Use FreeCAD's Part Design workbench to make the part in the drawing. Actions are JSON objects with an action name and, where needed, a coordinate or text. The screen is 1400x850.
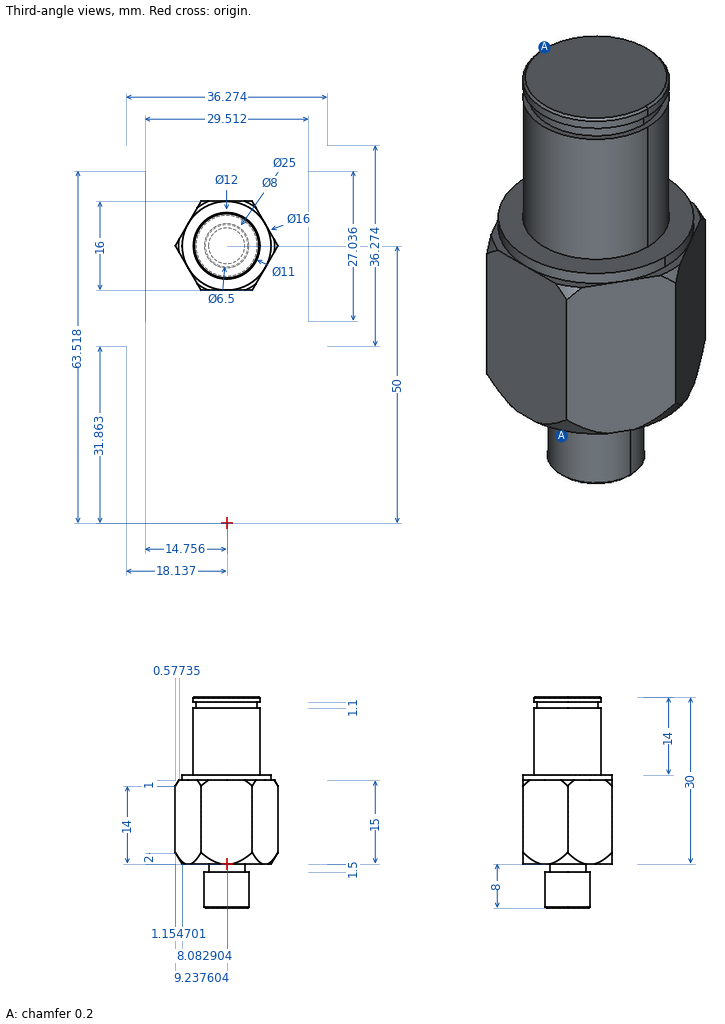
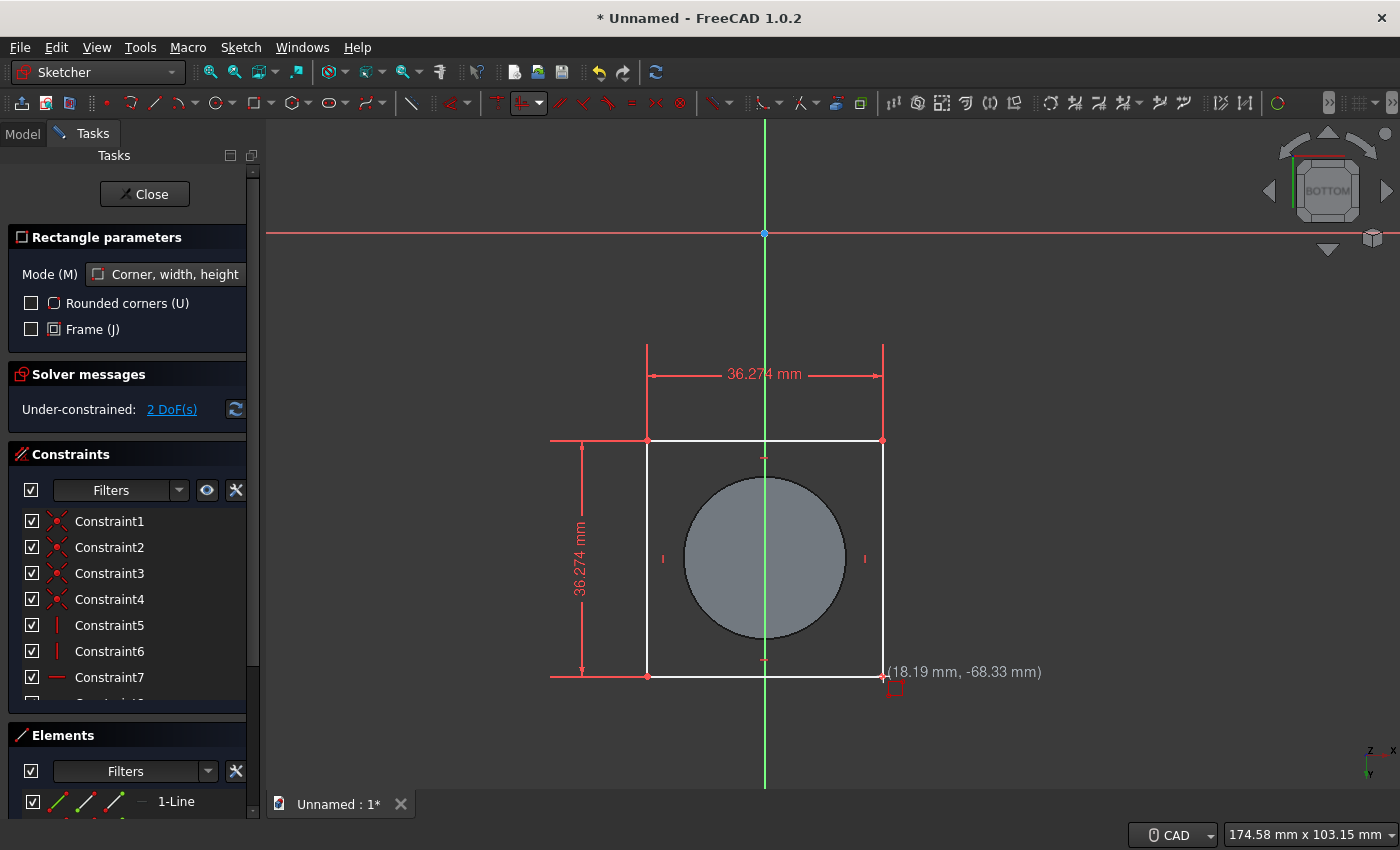
{"action": "left_click", "coordinate": [292, 104]}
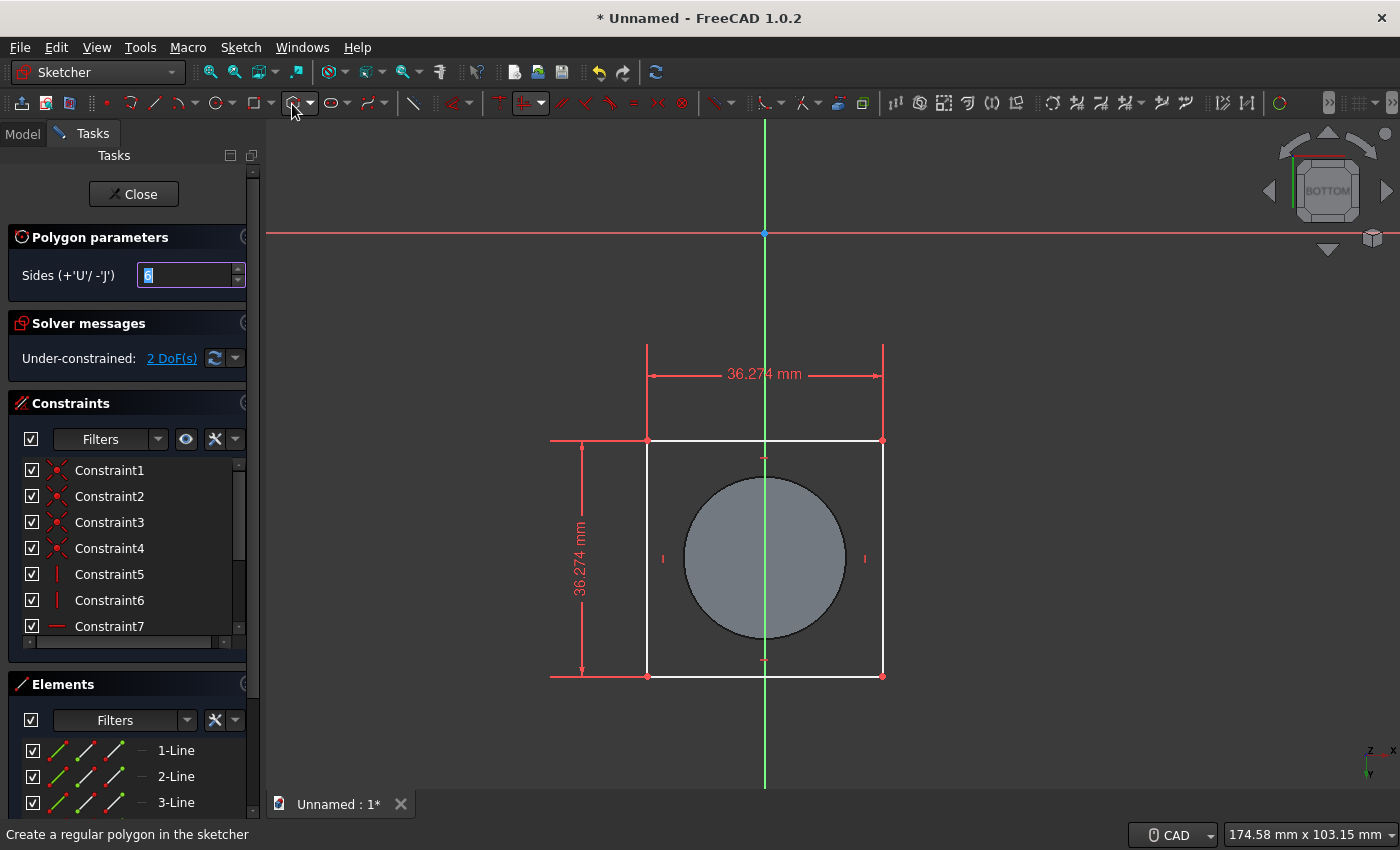
{"action": "left_click", "coordinate": [765, 558]}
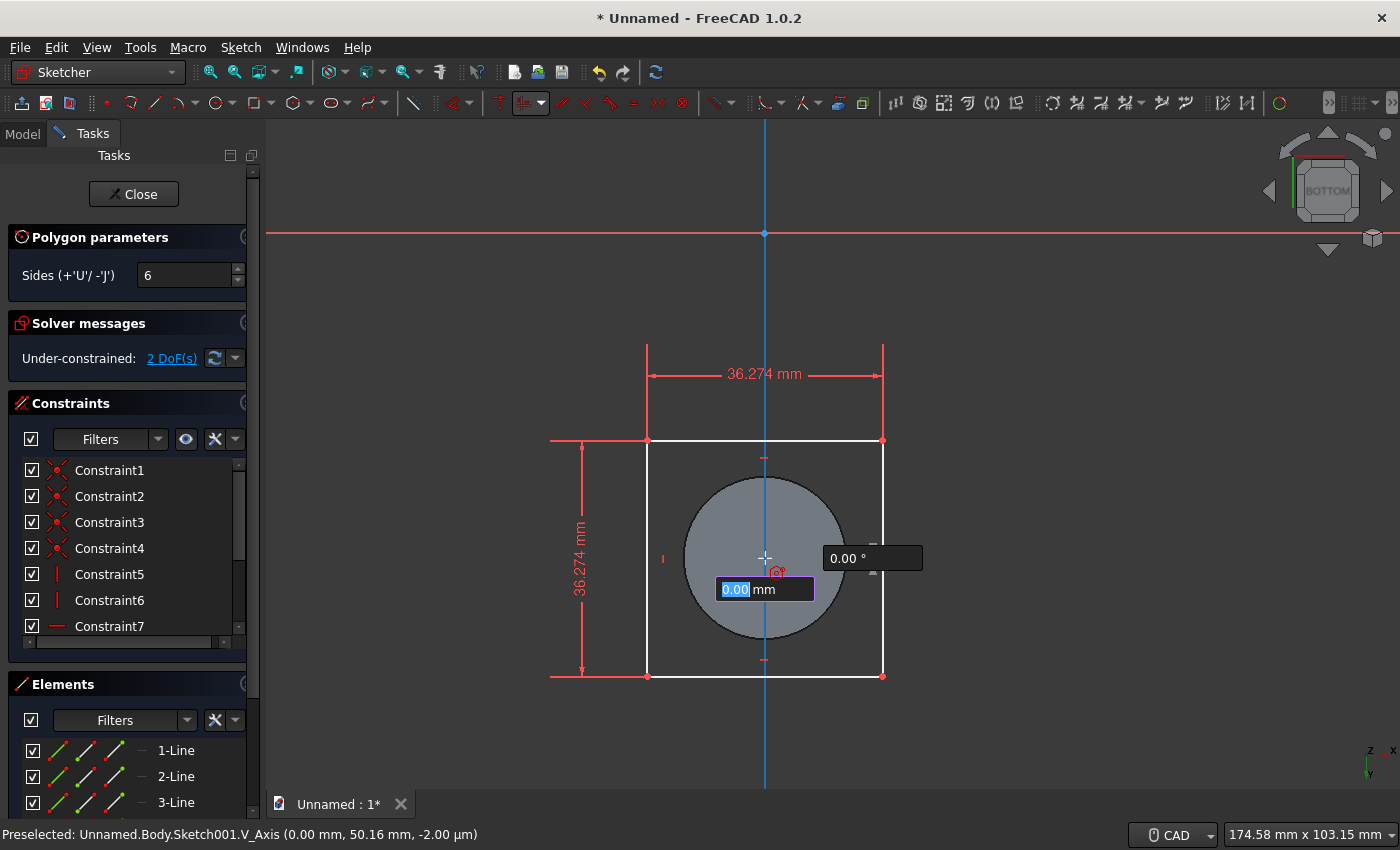
{"action": "left_click", "coordinate": [825, 558]}
{"action": "right_click", "coordinate": [825, 558]}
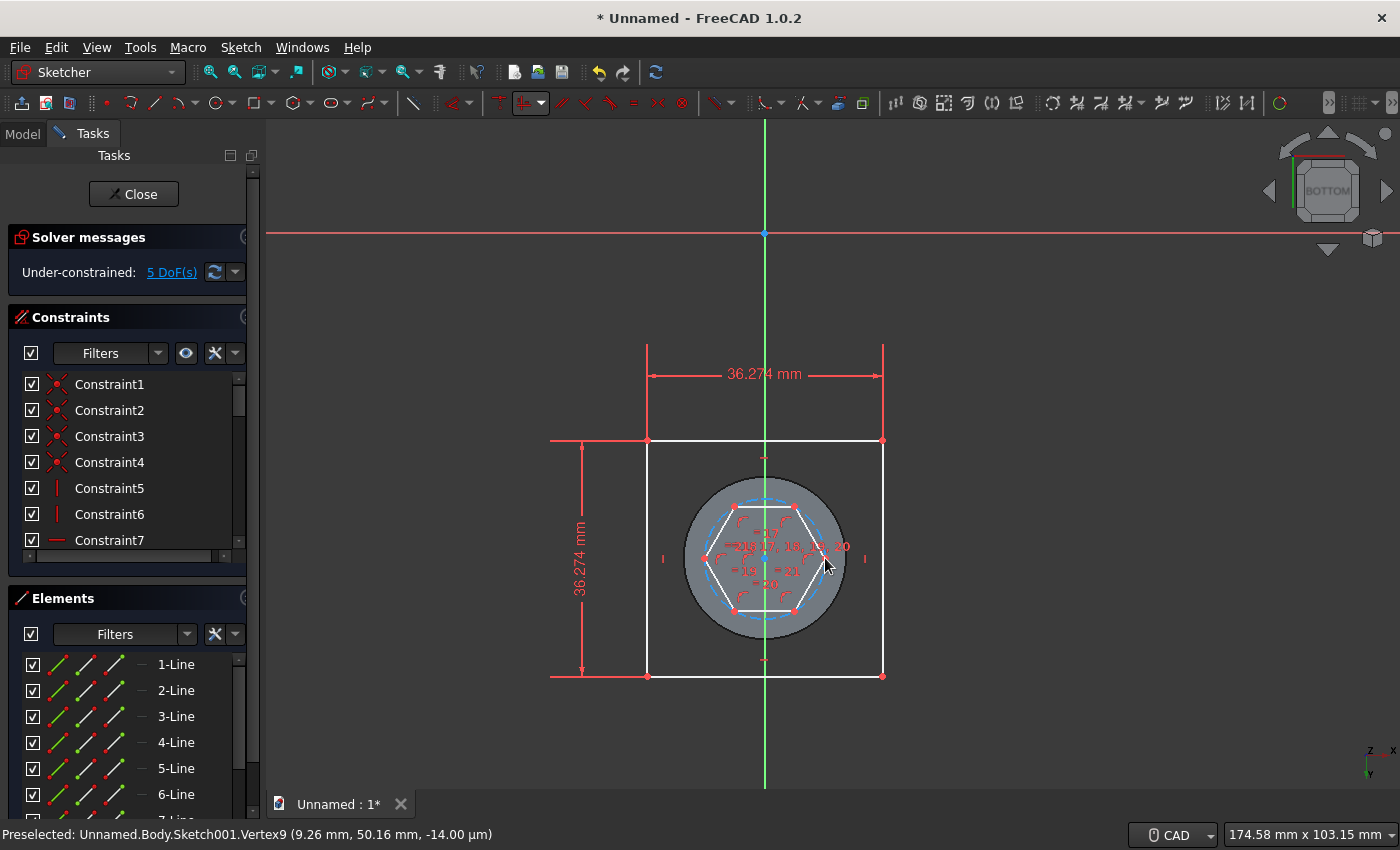
{"action": "scroll", "coordinate": [765, 507], "scroll_direction": "up", "scroll_amount": 3}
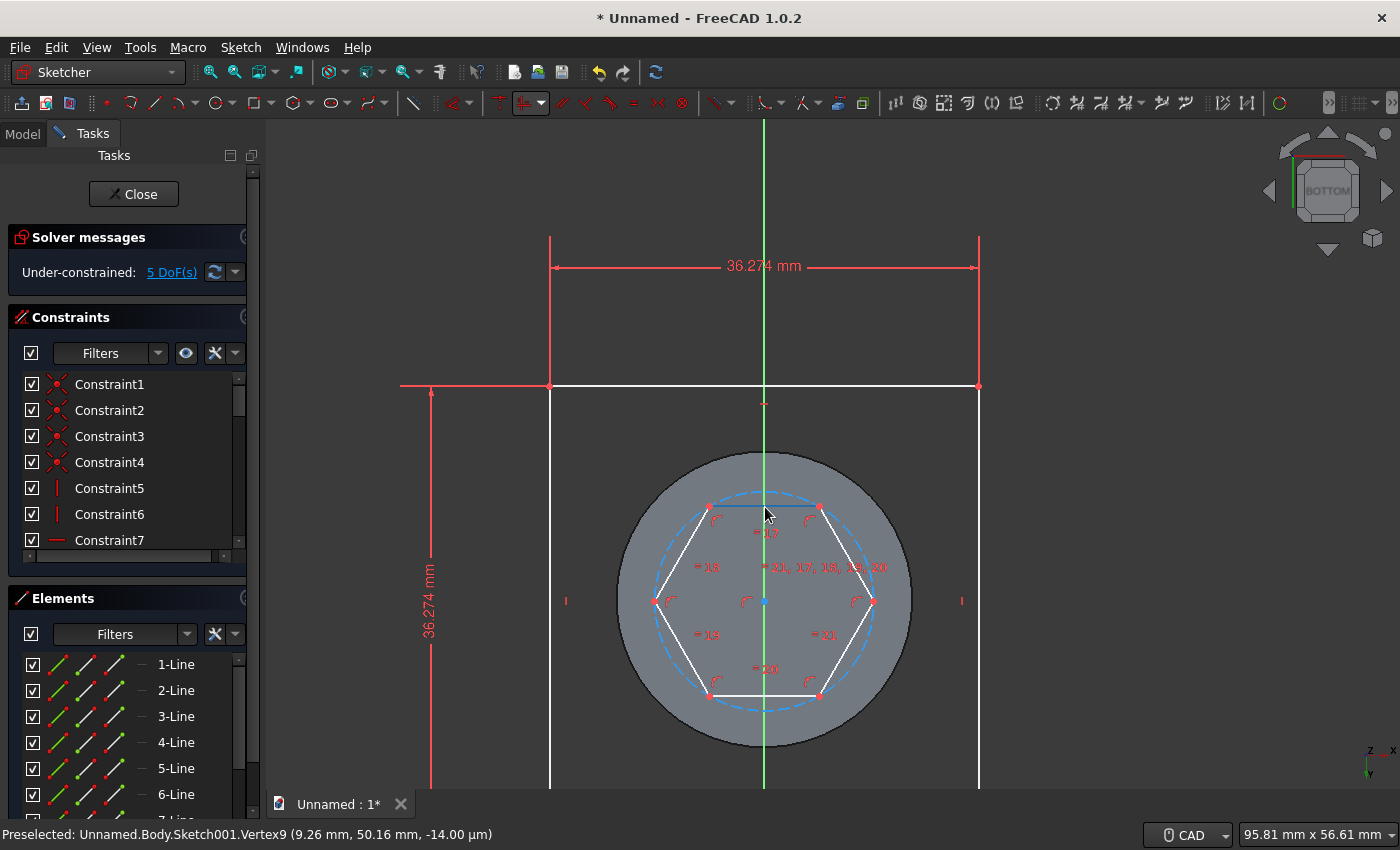
{"action": "left_click", "coordinate": [764, 506]}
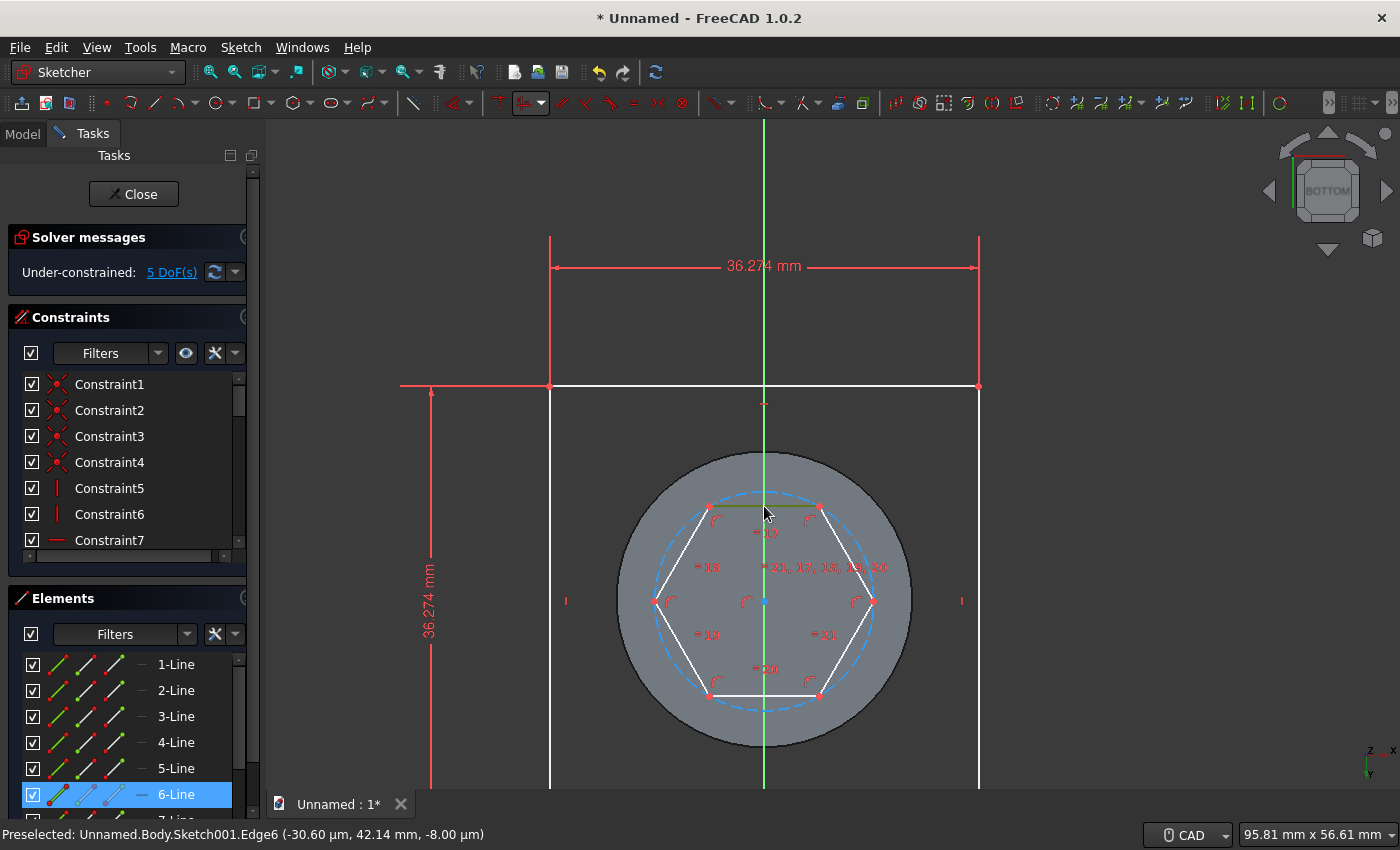
{"action": "key", "text": "h"}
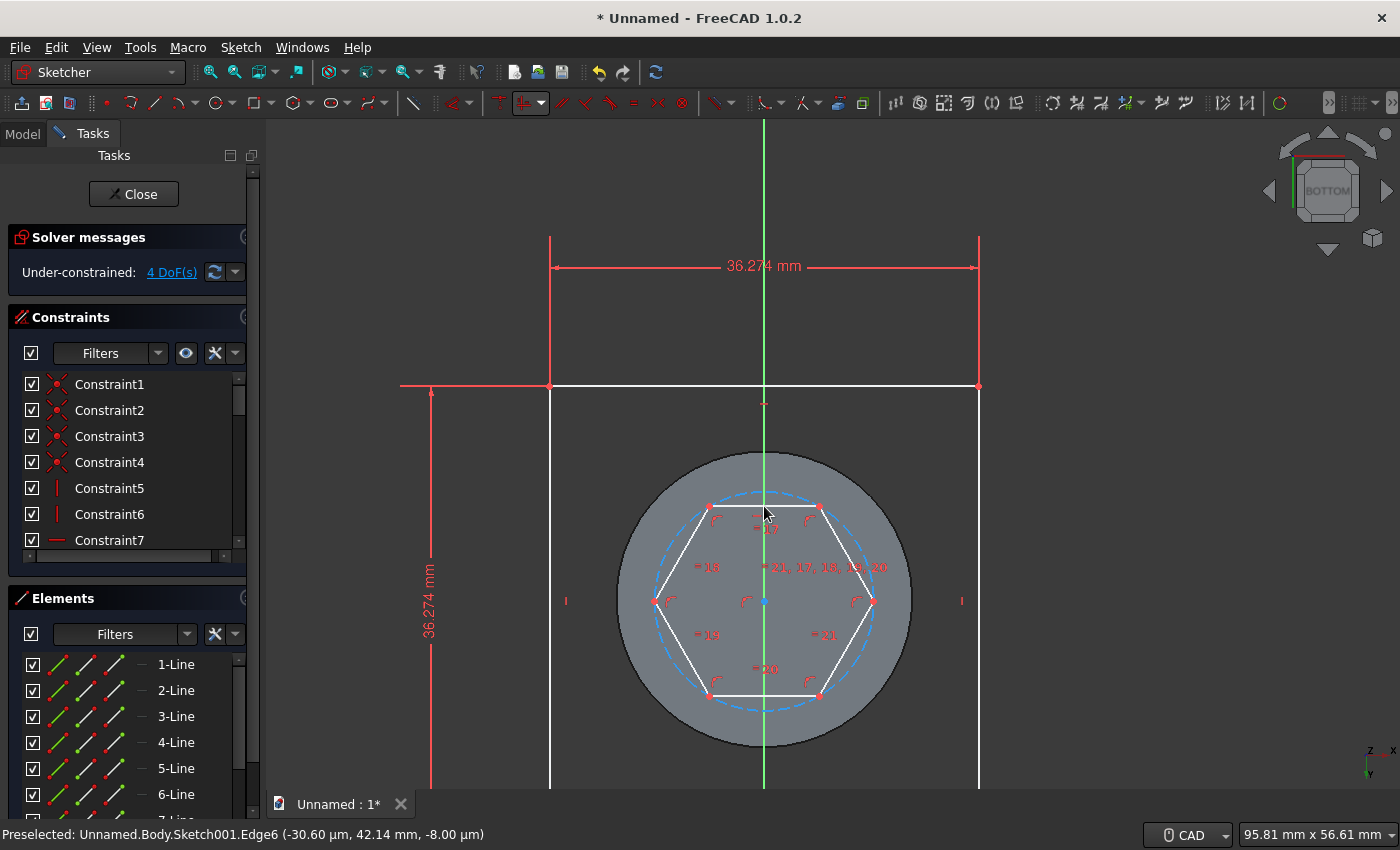
{"action": "left_click", "coordinate": [452, 104]}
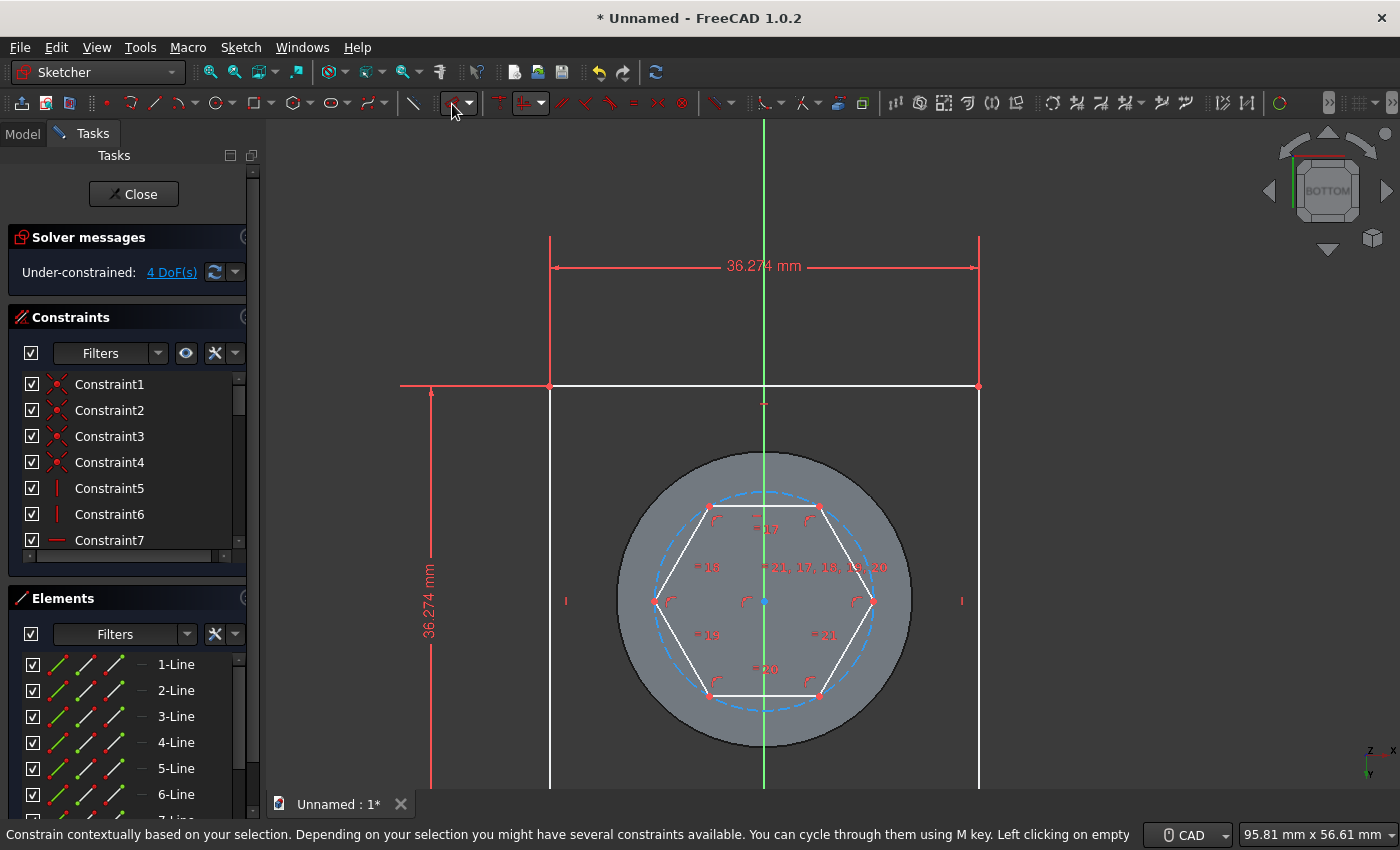
{"action": "left_click", "coordinate": [710, 696]}